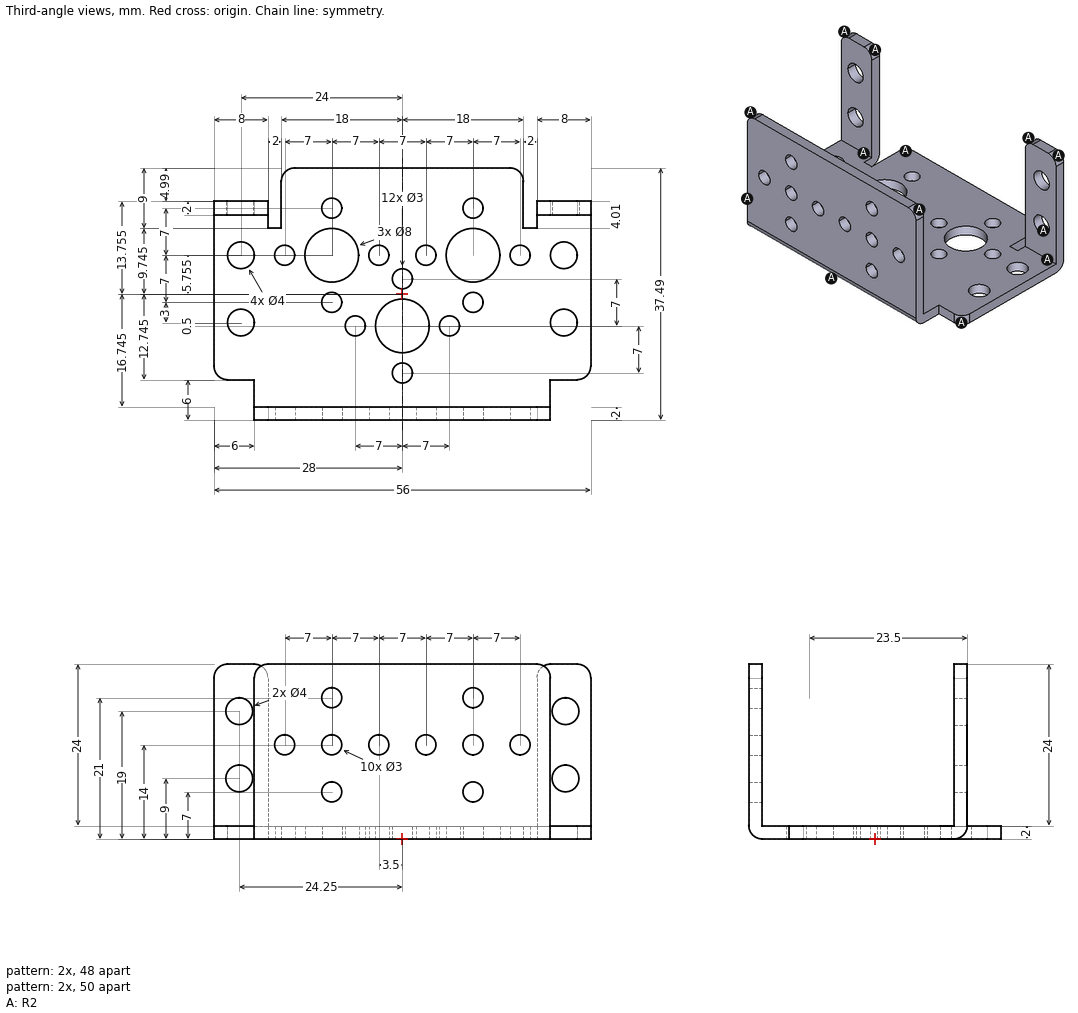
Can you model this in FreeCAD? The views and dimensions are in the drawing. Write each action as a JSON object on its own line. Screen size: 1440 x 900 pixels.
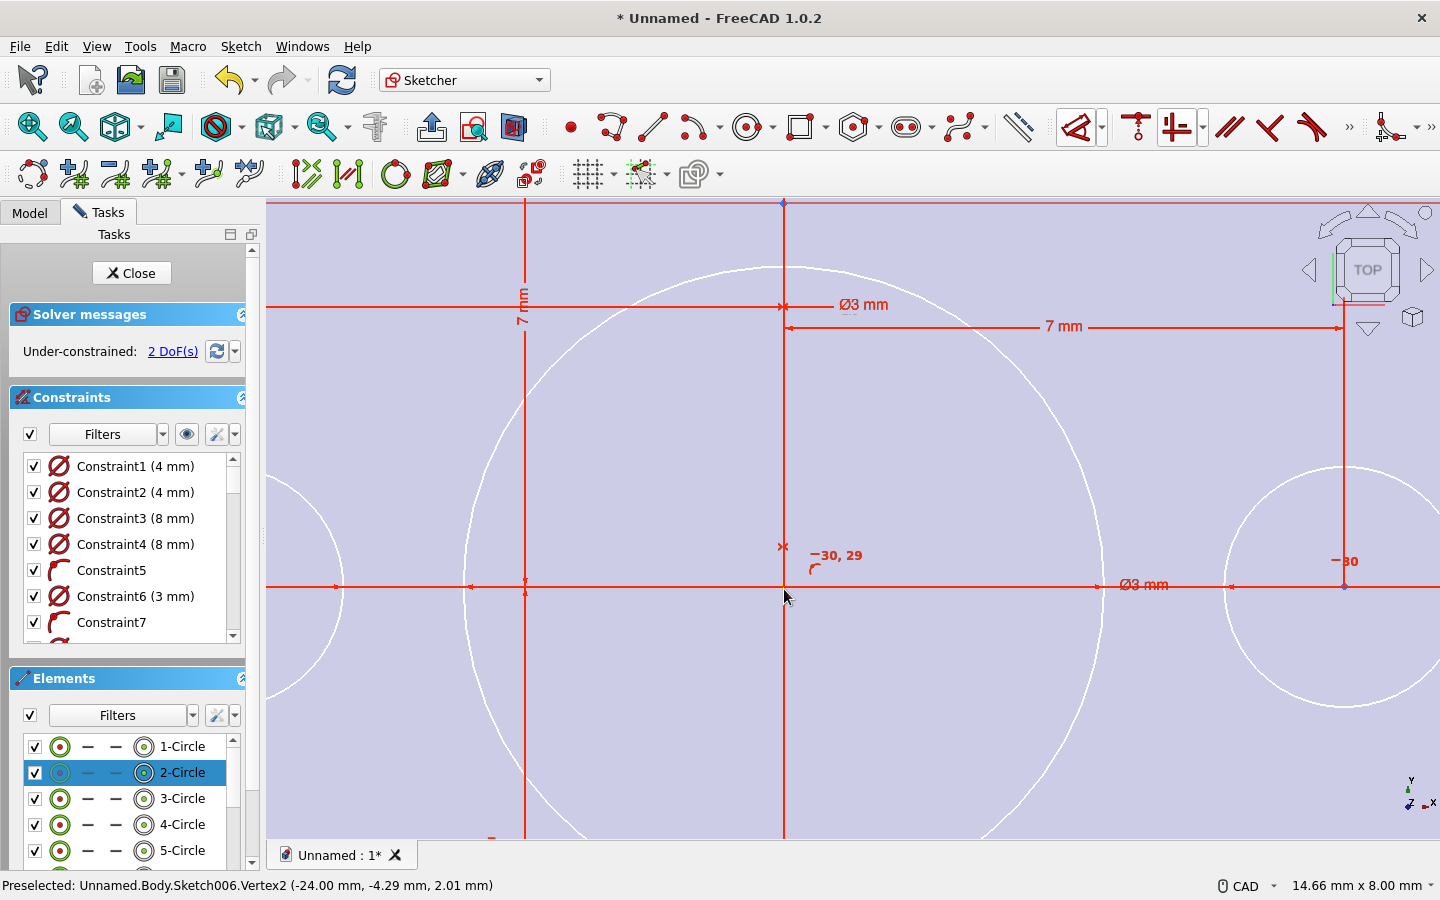
{"action": "left_click", "coordinate": [784, 587]}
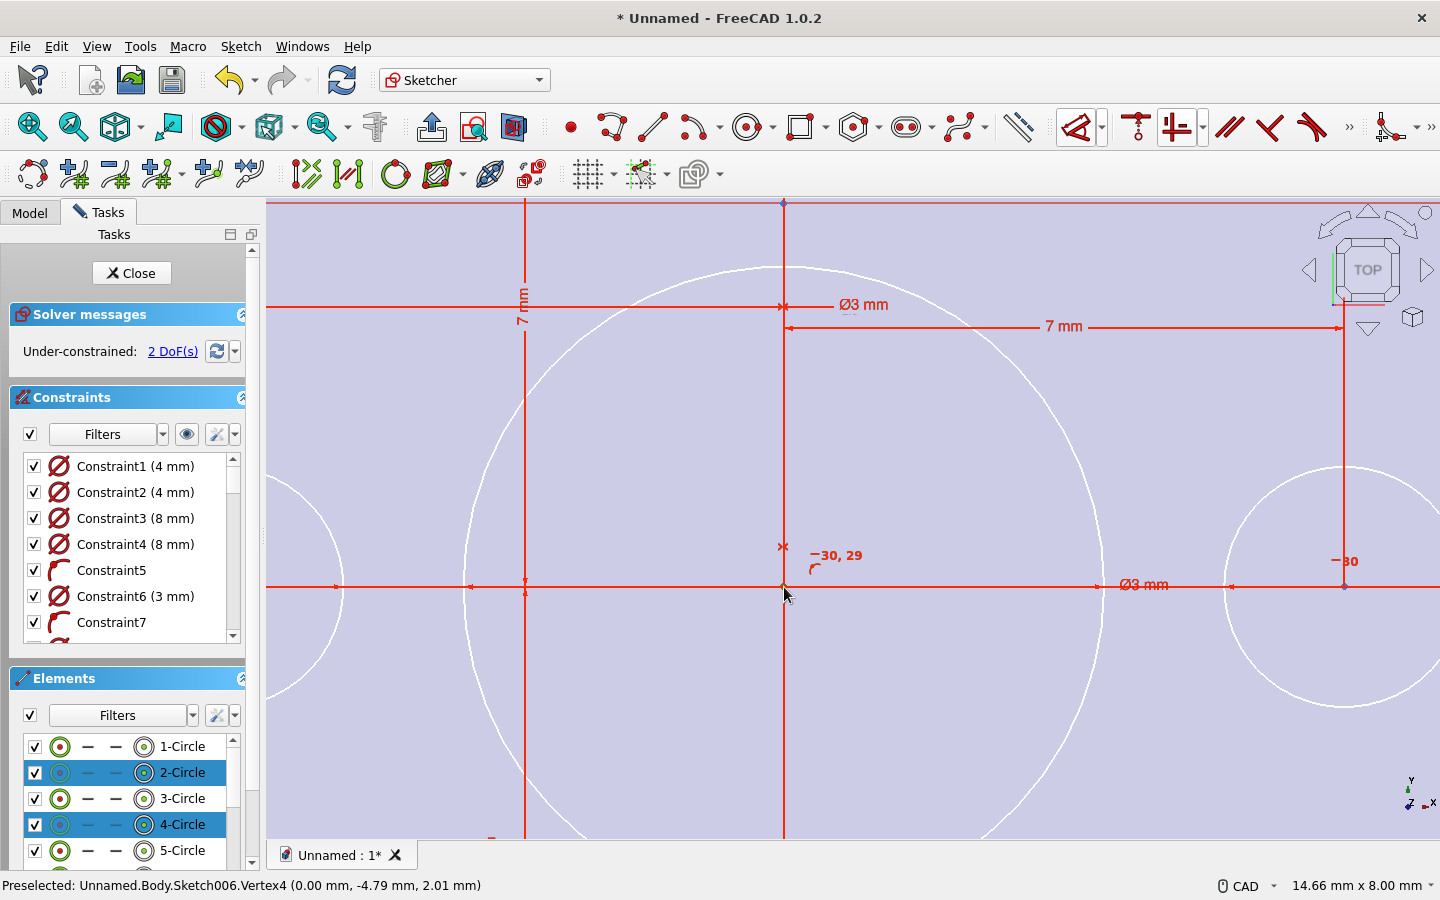
{"action": "key", "text": "i"}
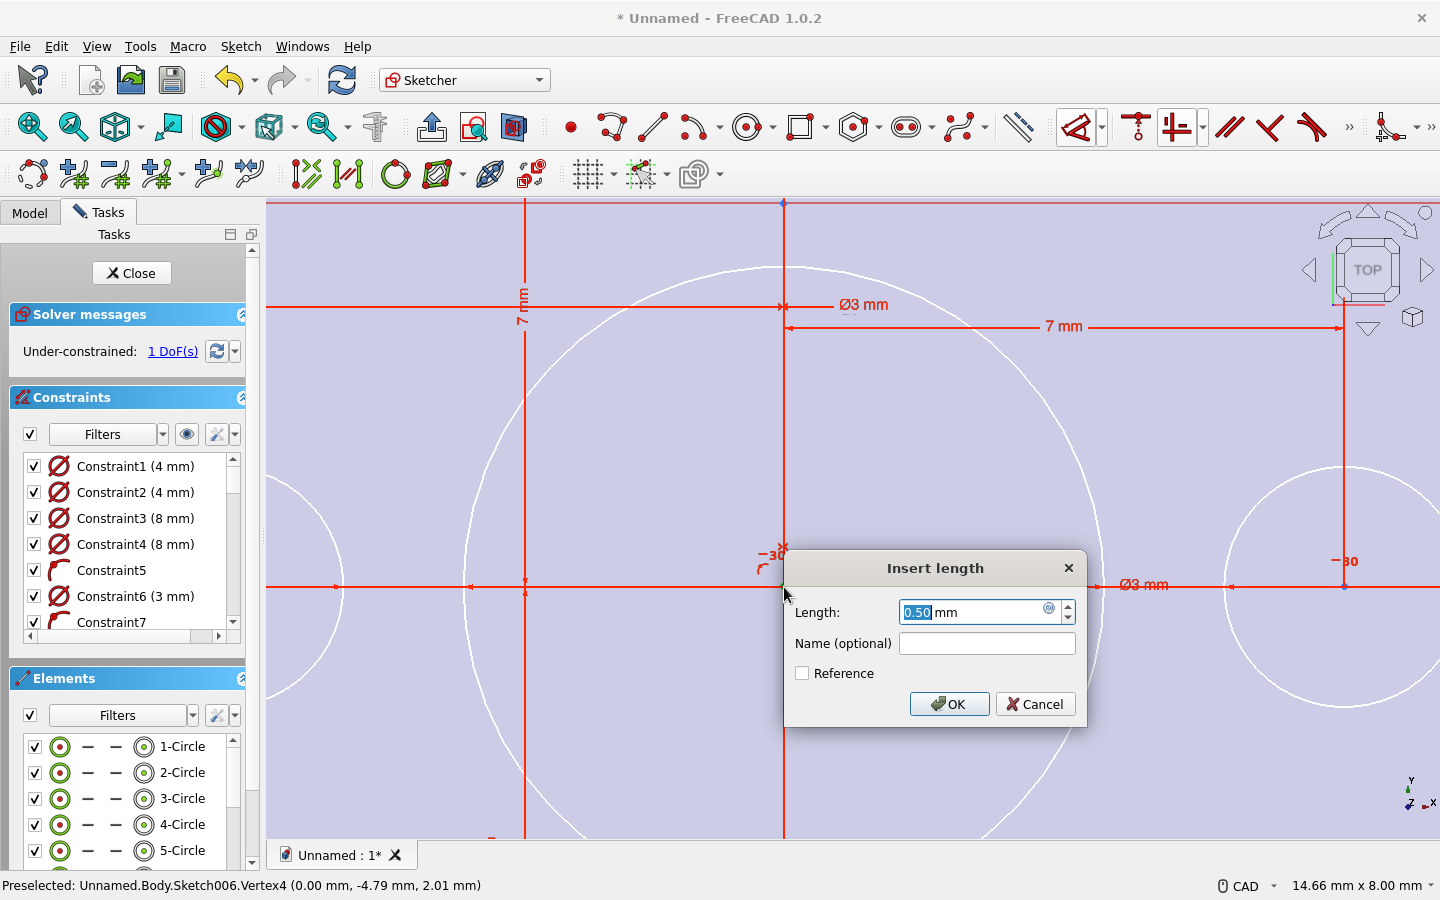
{"action": "type", "text": "0.5"}
{"action": "key", "text": "Return"}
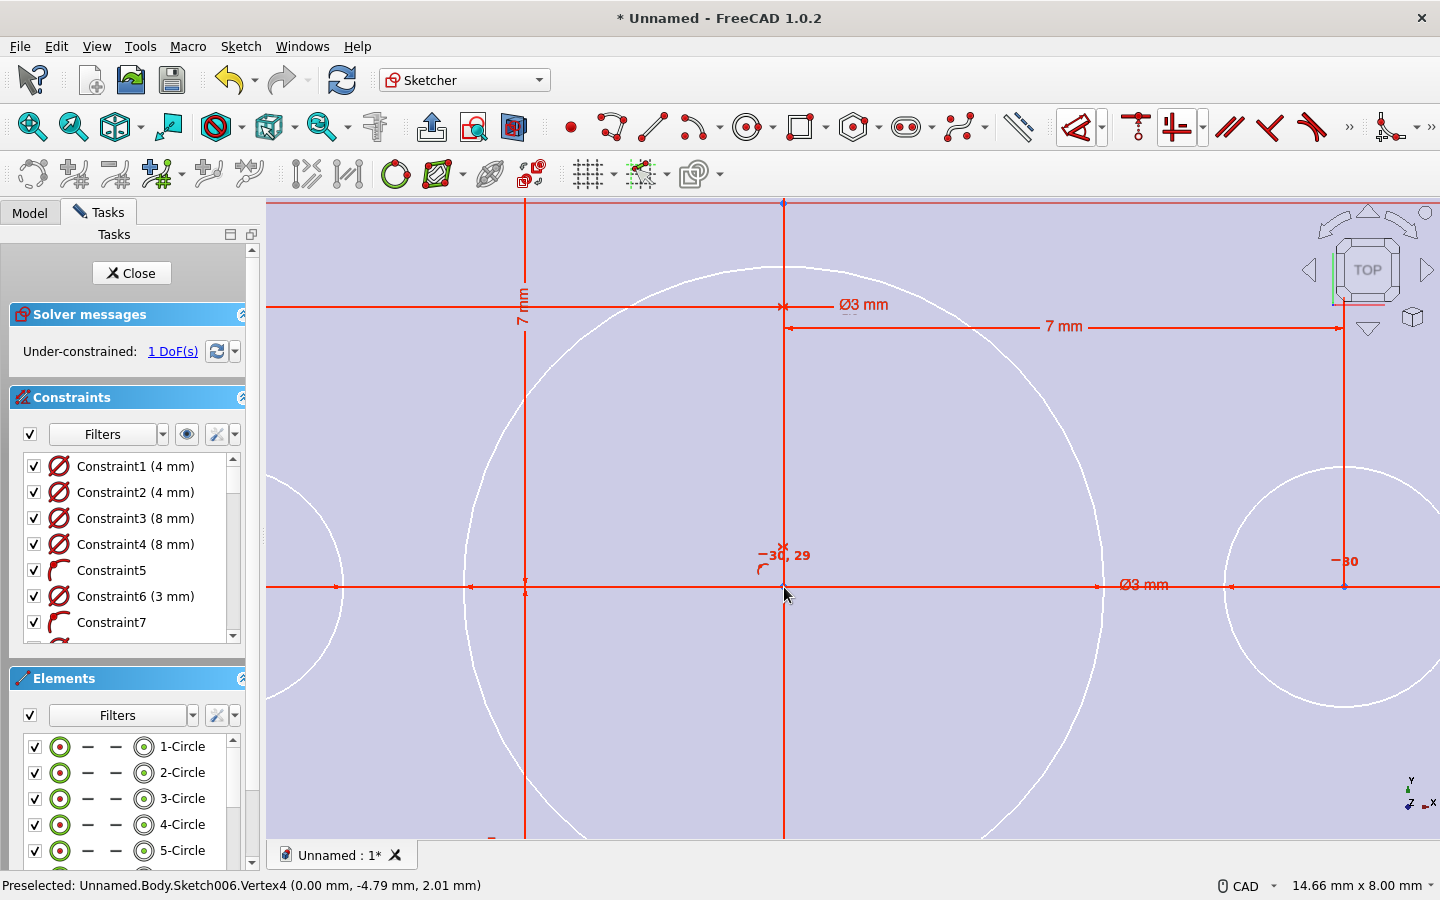
{"action": "scroll", "coordinate": [785, 589], "scroll_direction": "down", "scroll_amount": 9}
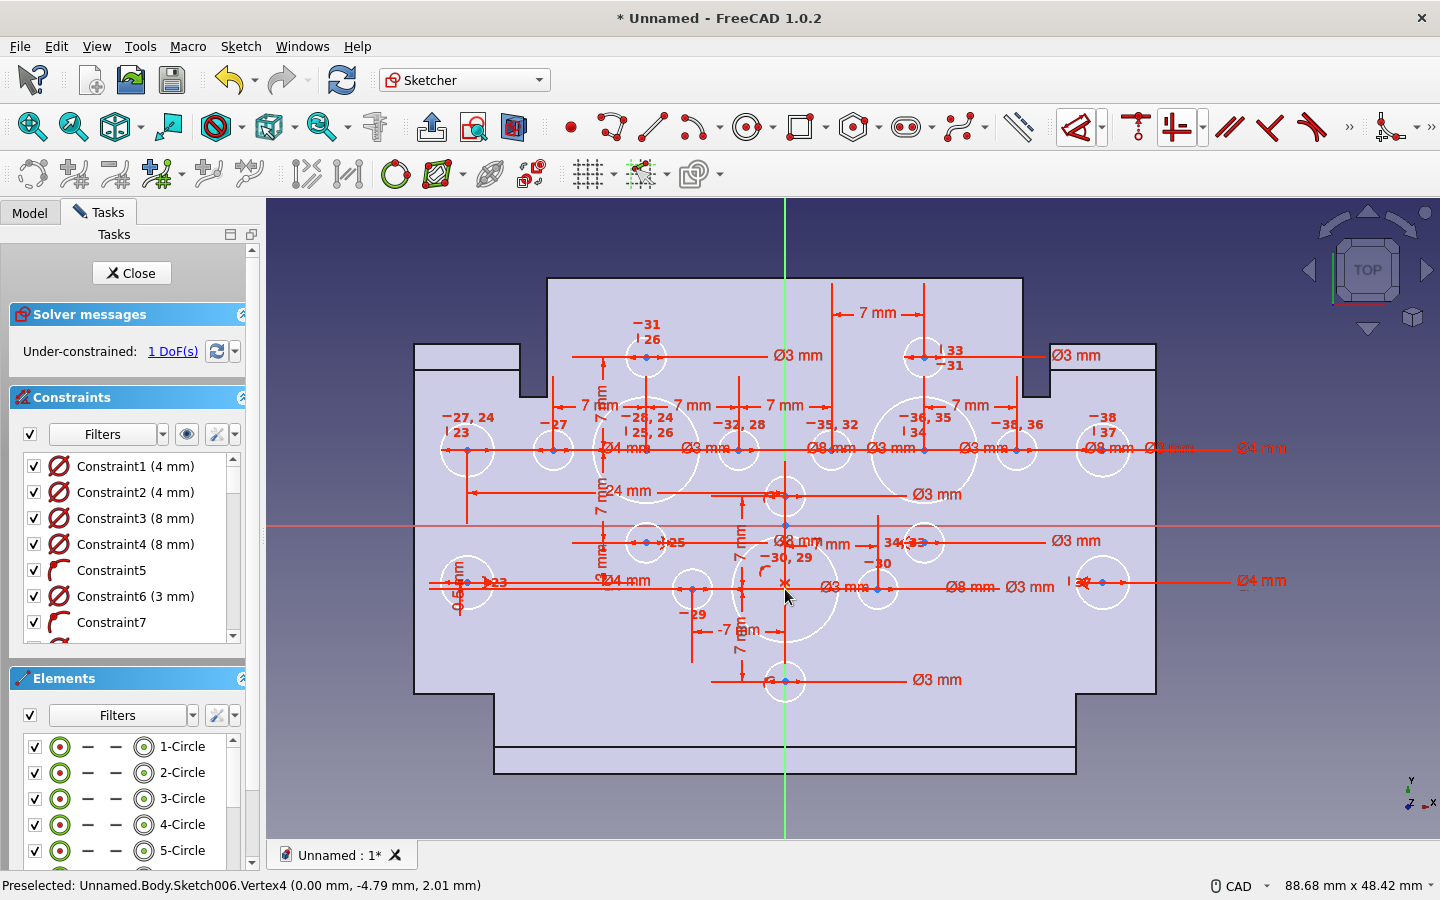
{"action": "left_click", "coordinate": [467, 450]}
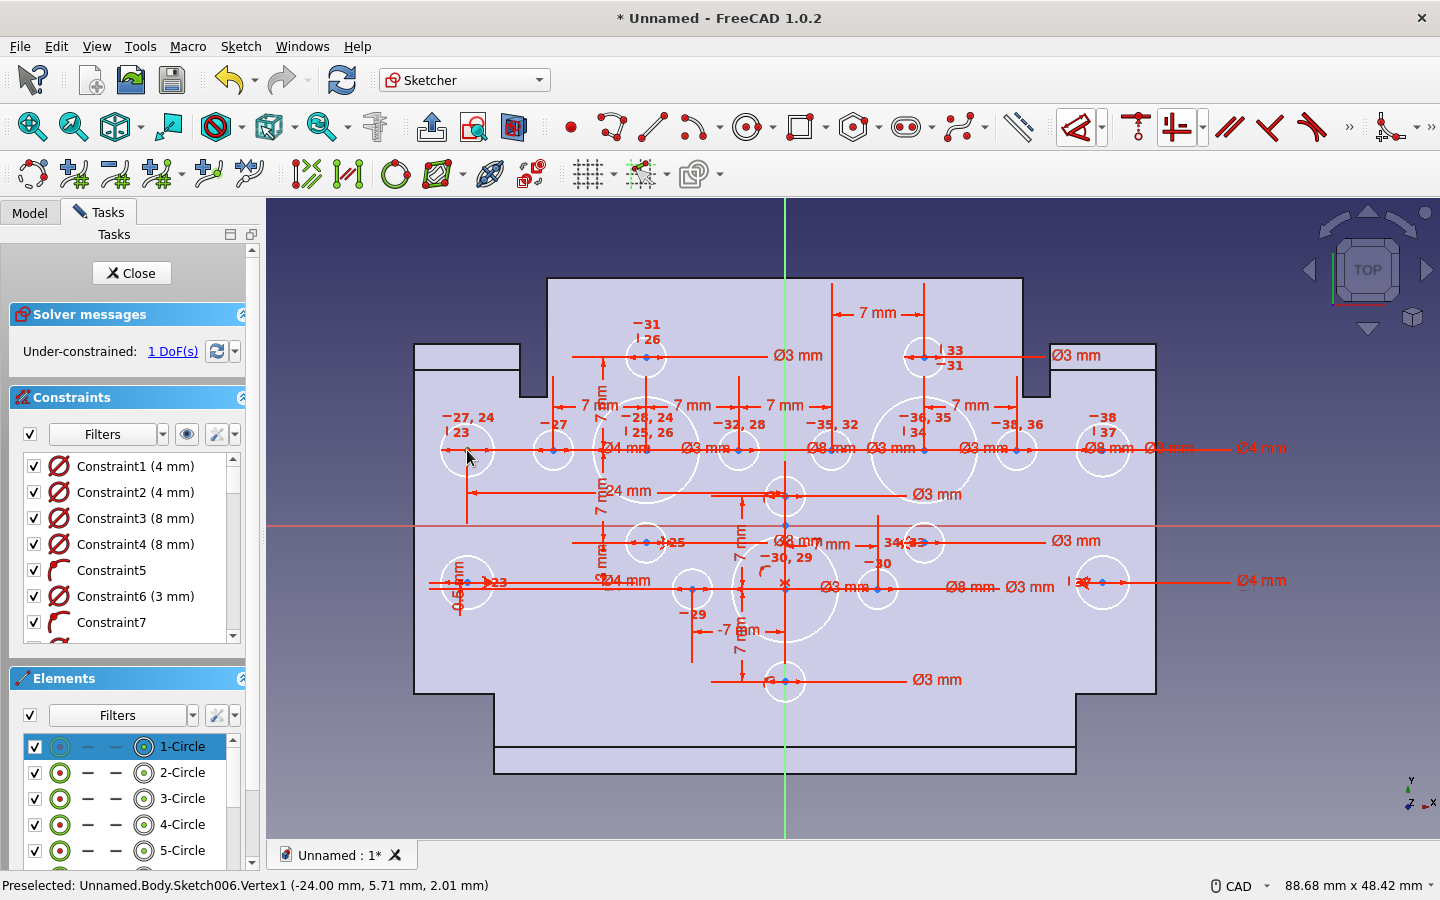
{"action": "key", "text": "i"}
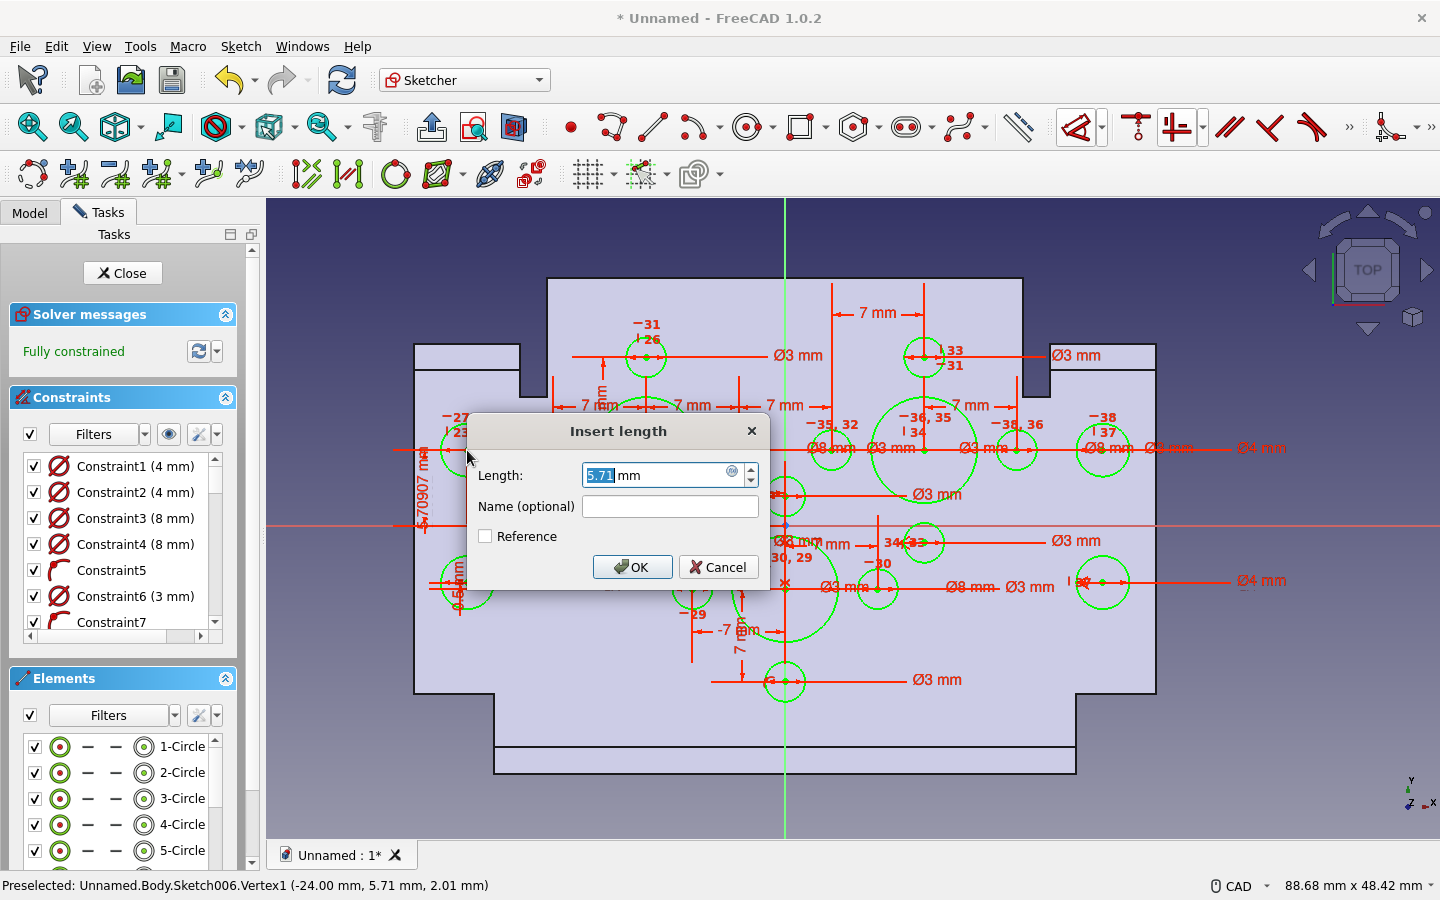
{"action": "type", "text": "5.755"}
{"action": "key", "text": "Return"}